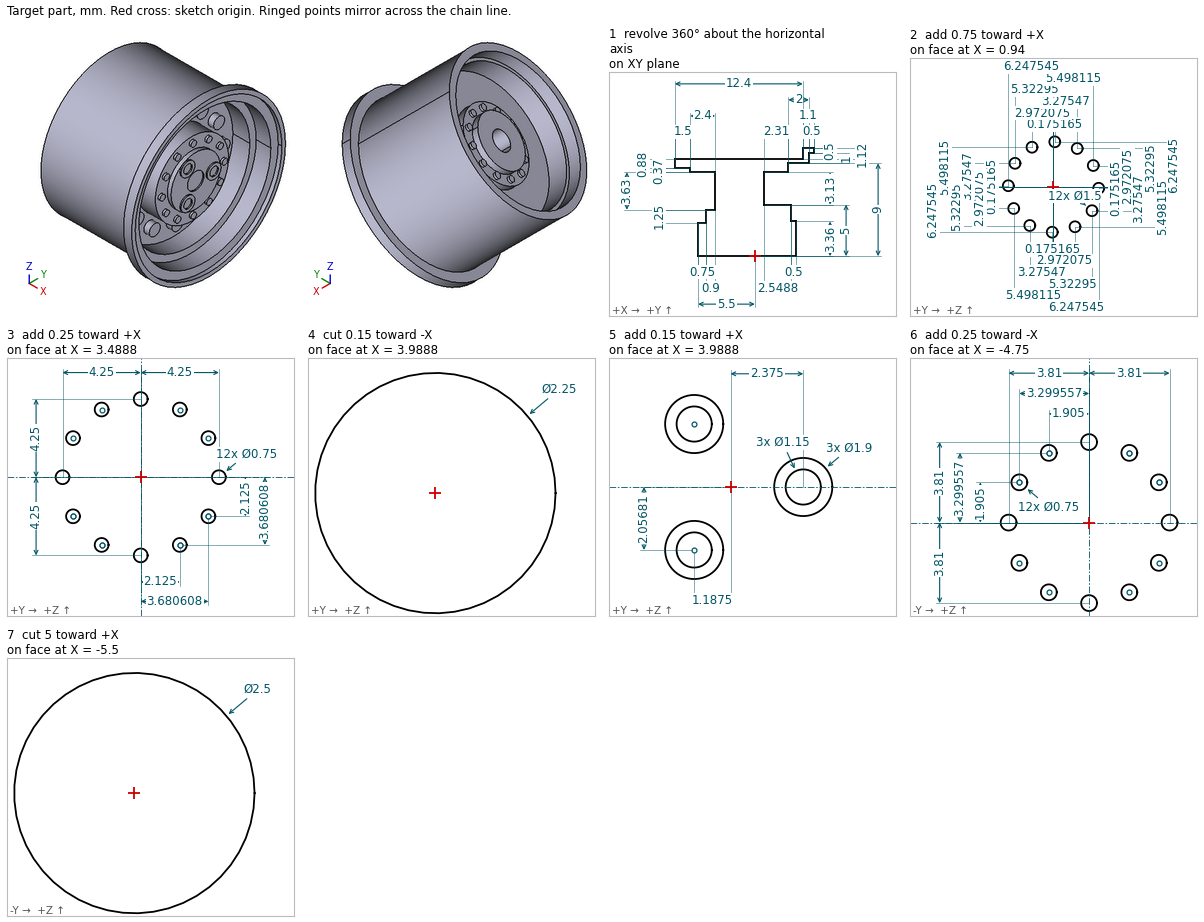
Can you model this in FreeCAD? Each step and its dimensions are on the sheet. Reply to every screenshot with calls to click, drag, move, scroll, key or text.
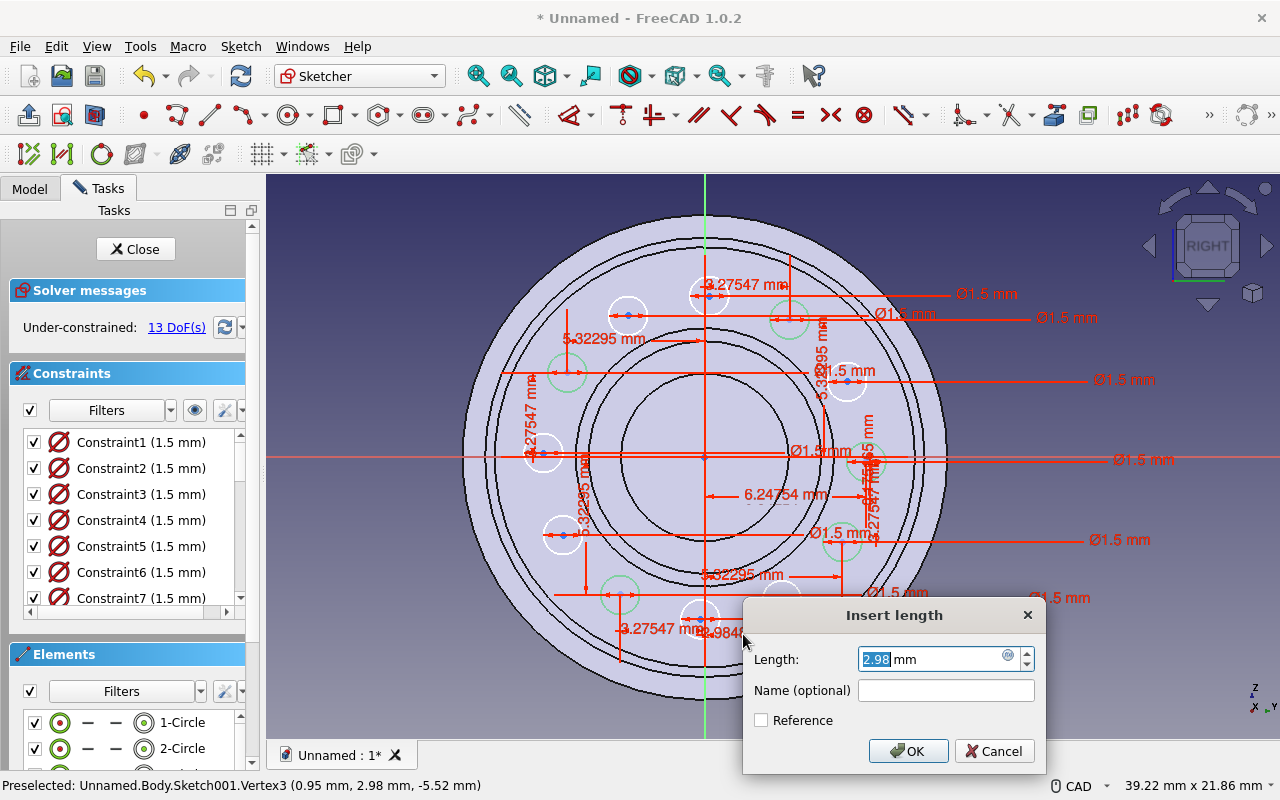
text(2.972075)
key(Return)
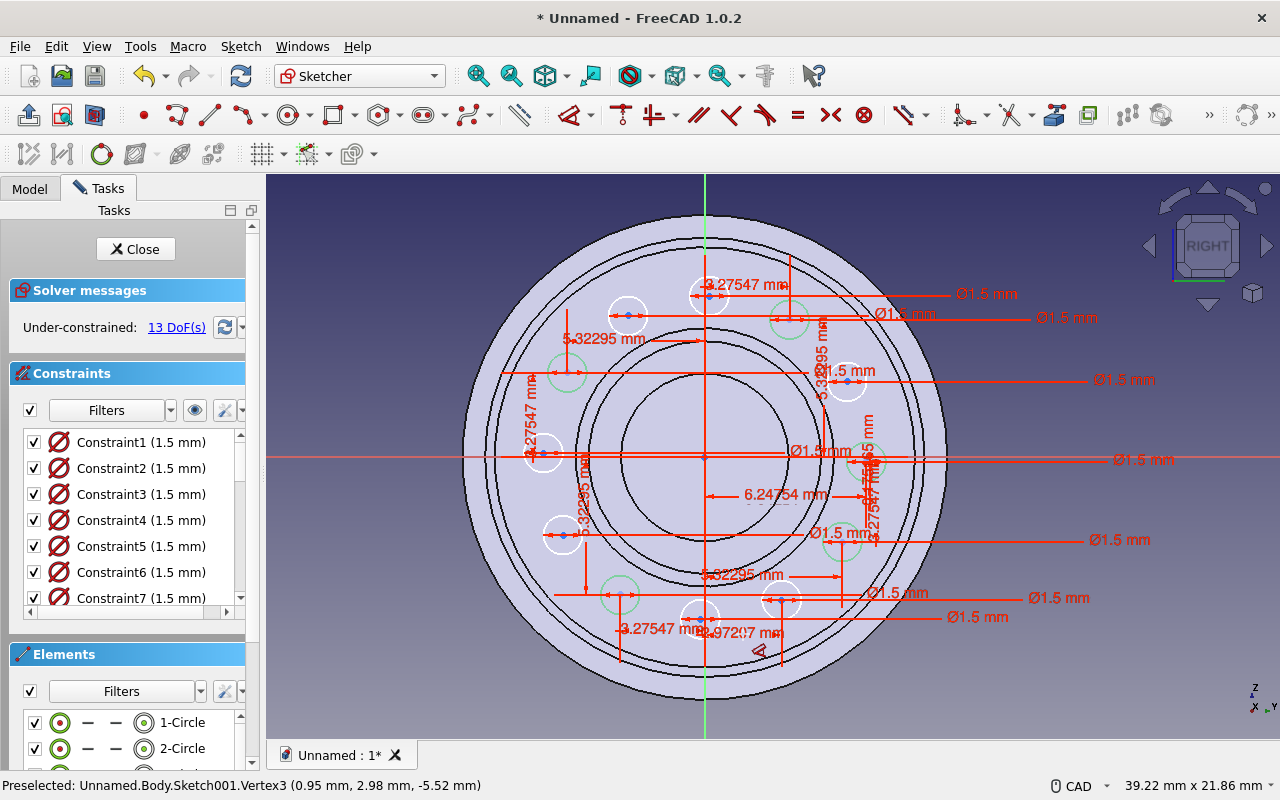
click(782, 600)
click(816, 562)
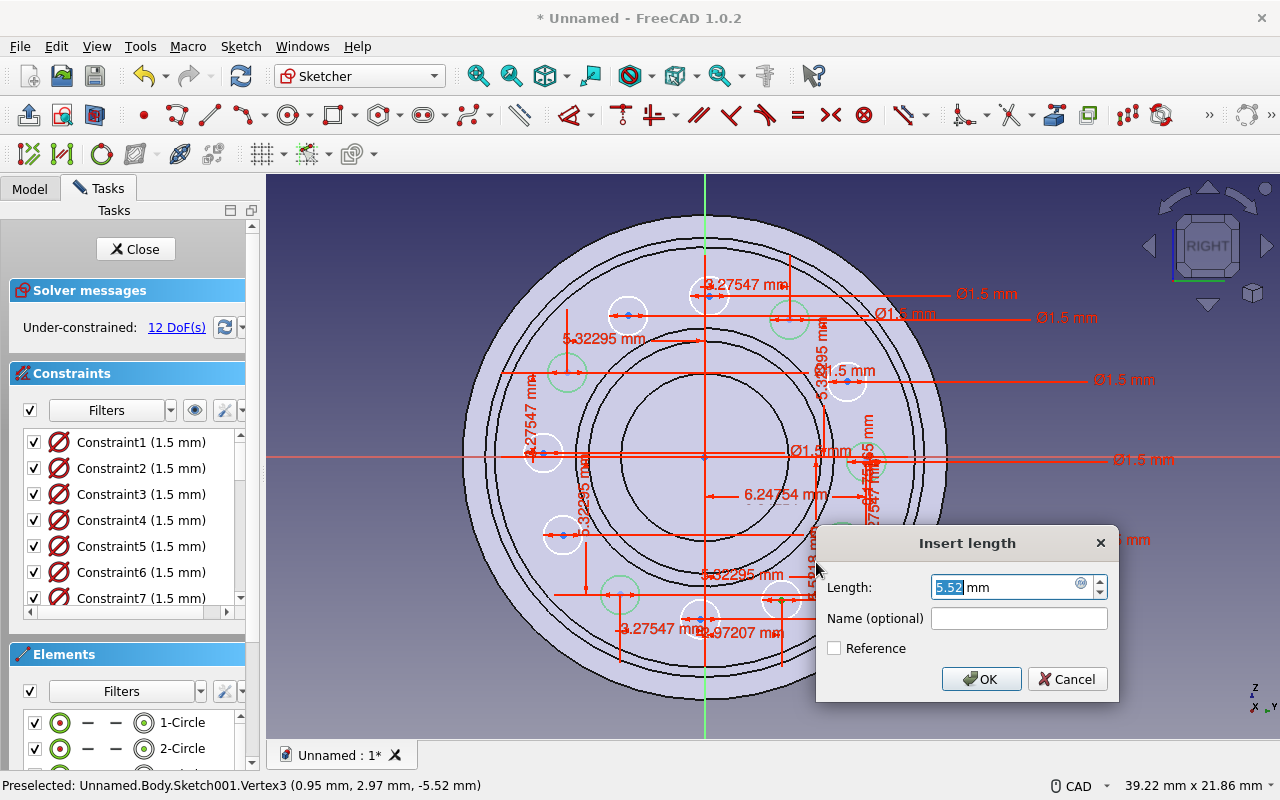
text(5.498115)
key(Return)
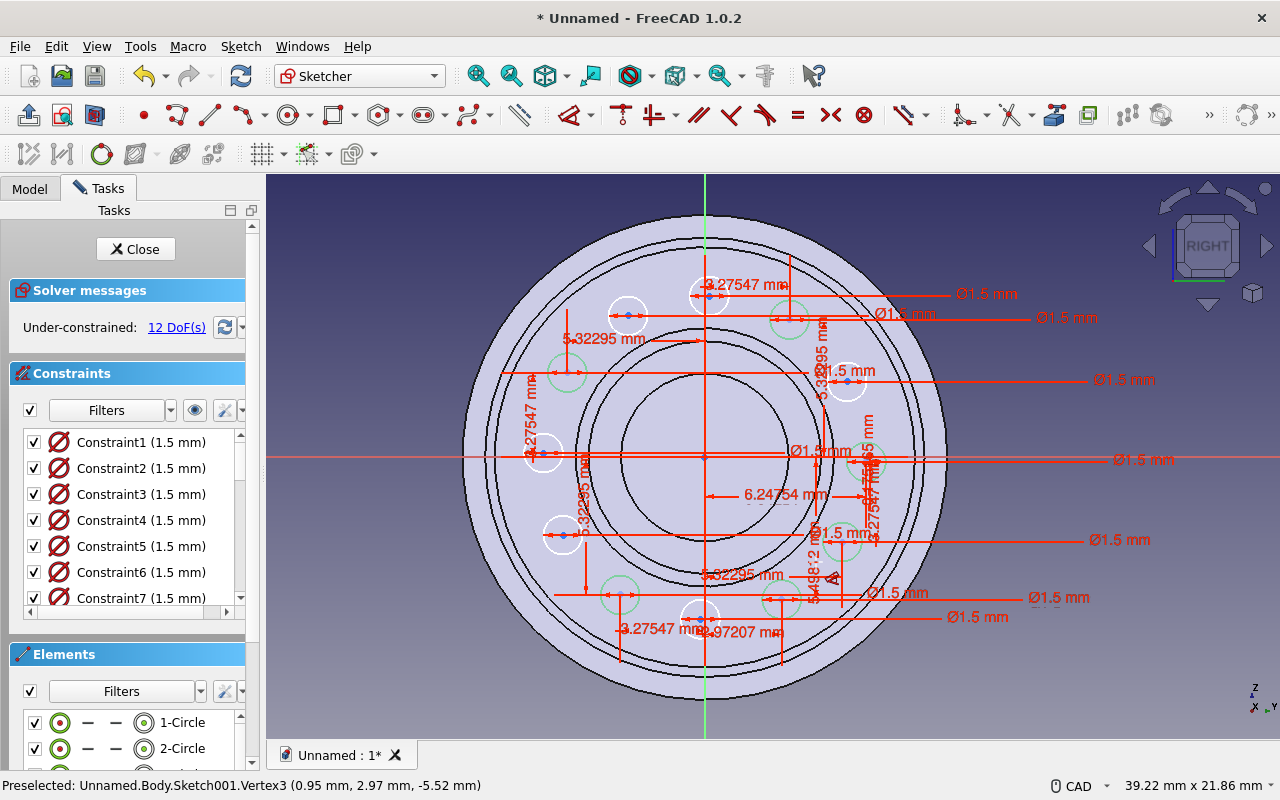
scroll(700, 619, up, 11)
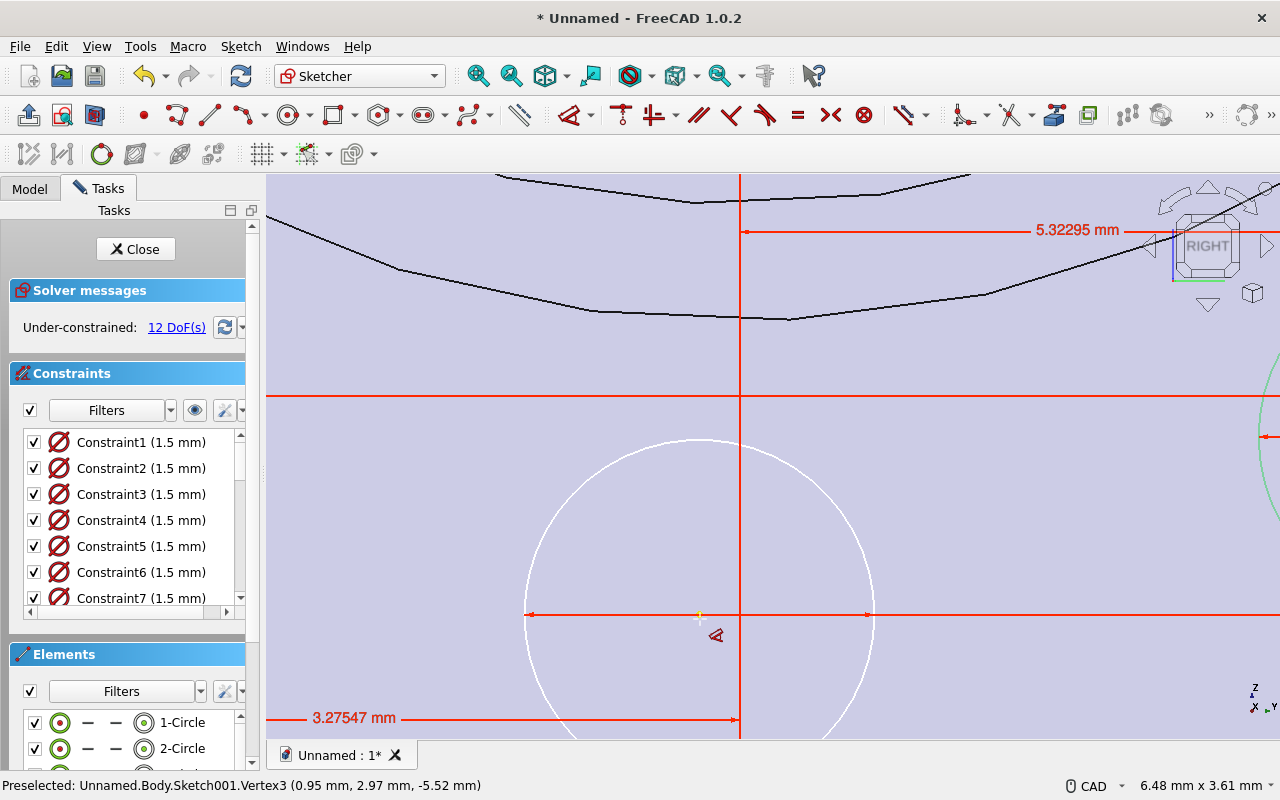
click(699, 615)
click(720, 649)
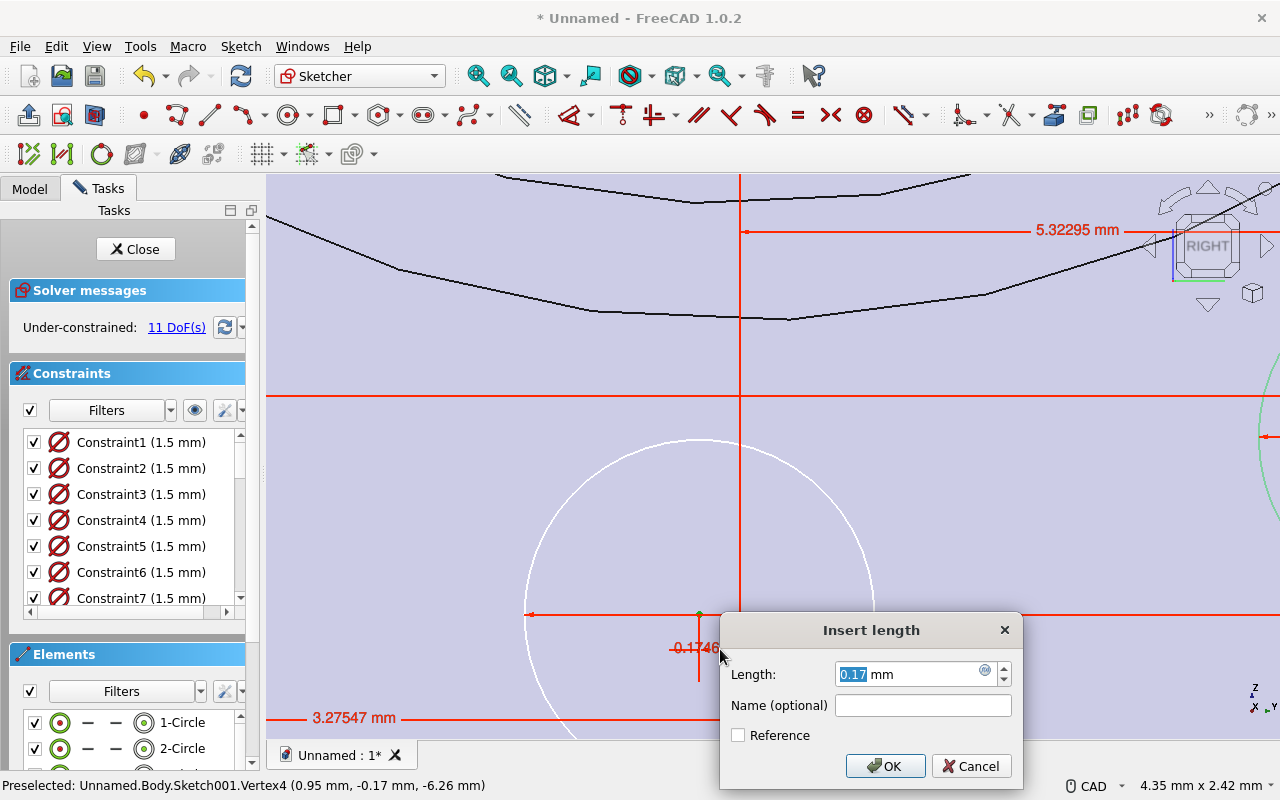
text(0.175165)
key(Return)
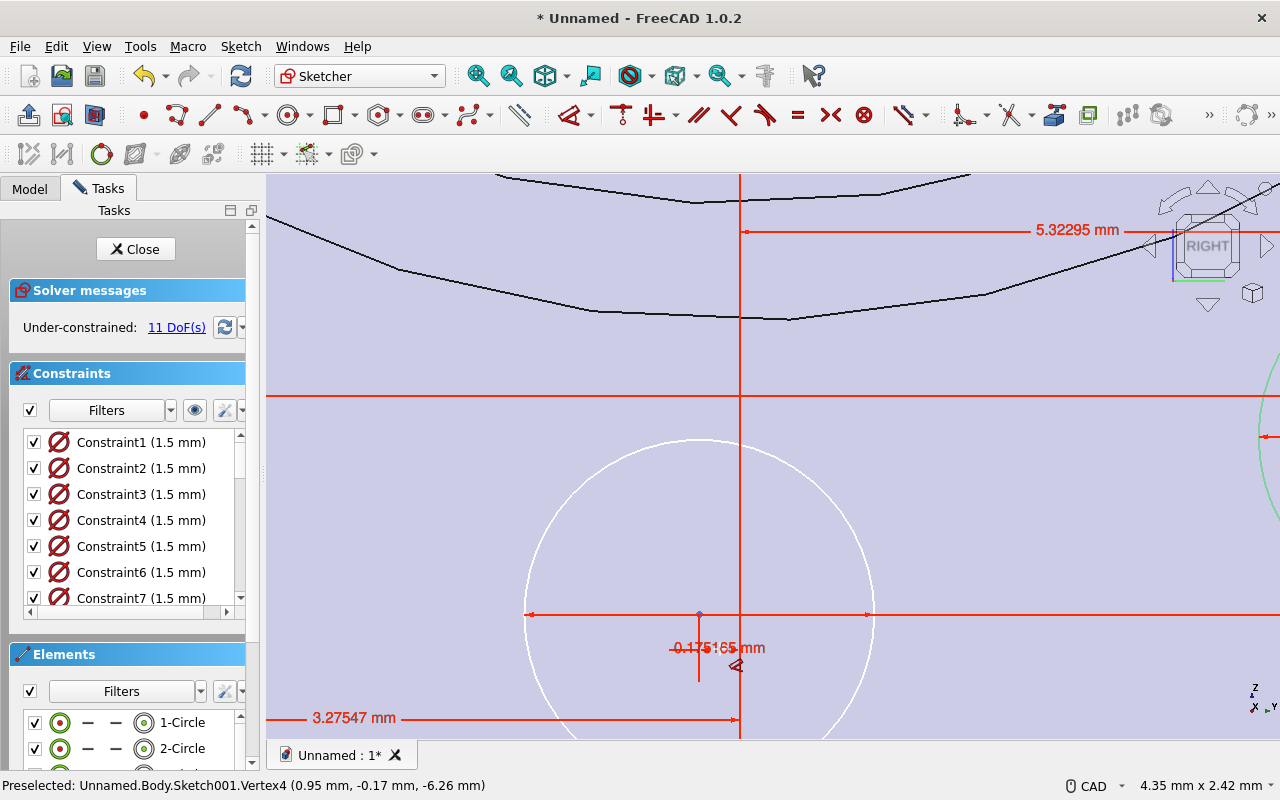
scroll(700, 619, down, 11)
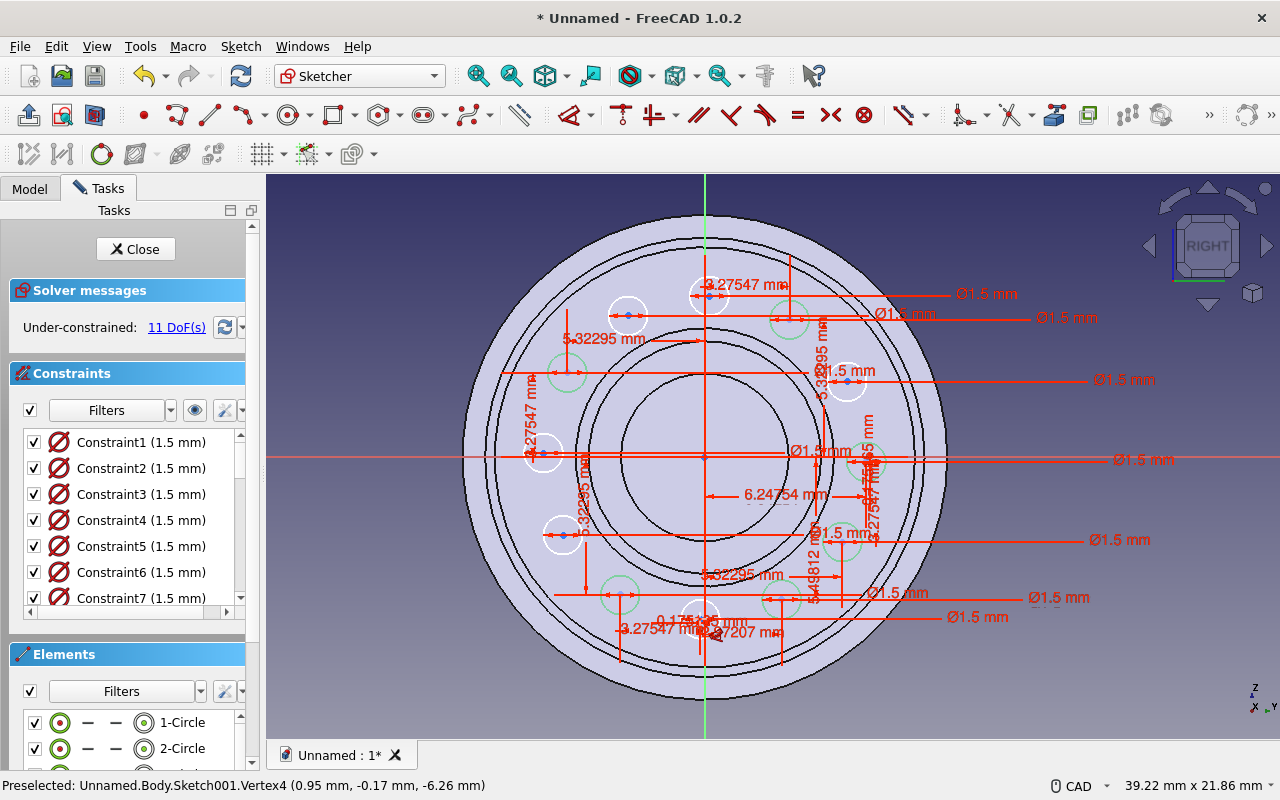
click(700, 619)
click(666, 538)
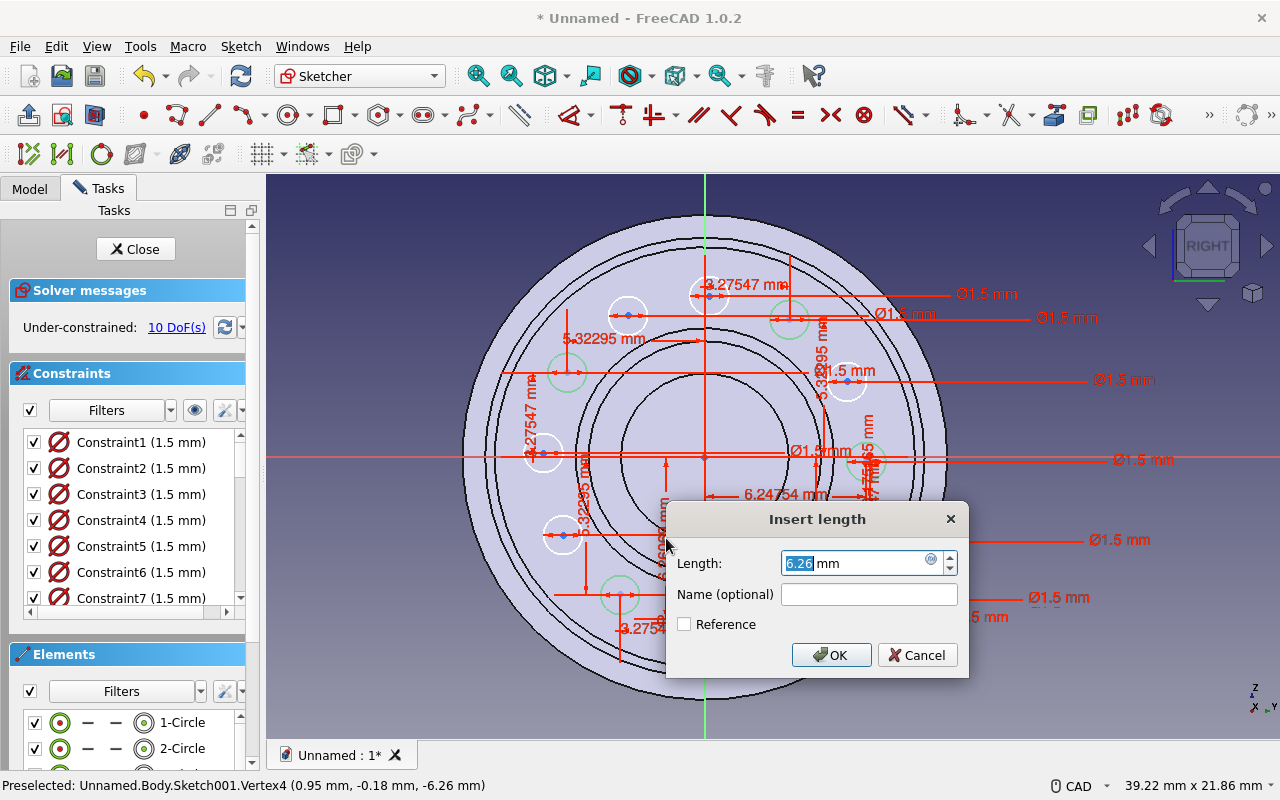
text(6.247545)
key(Return)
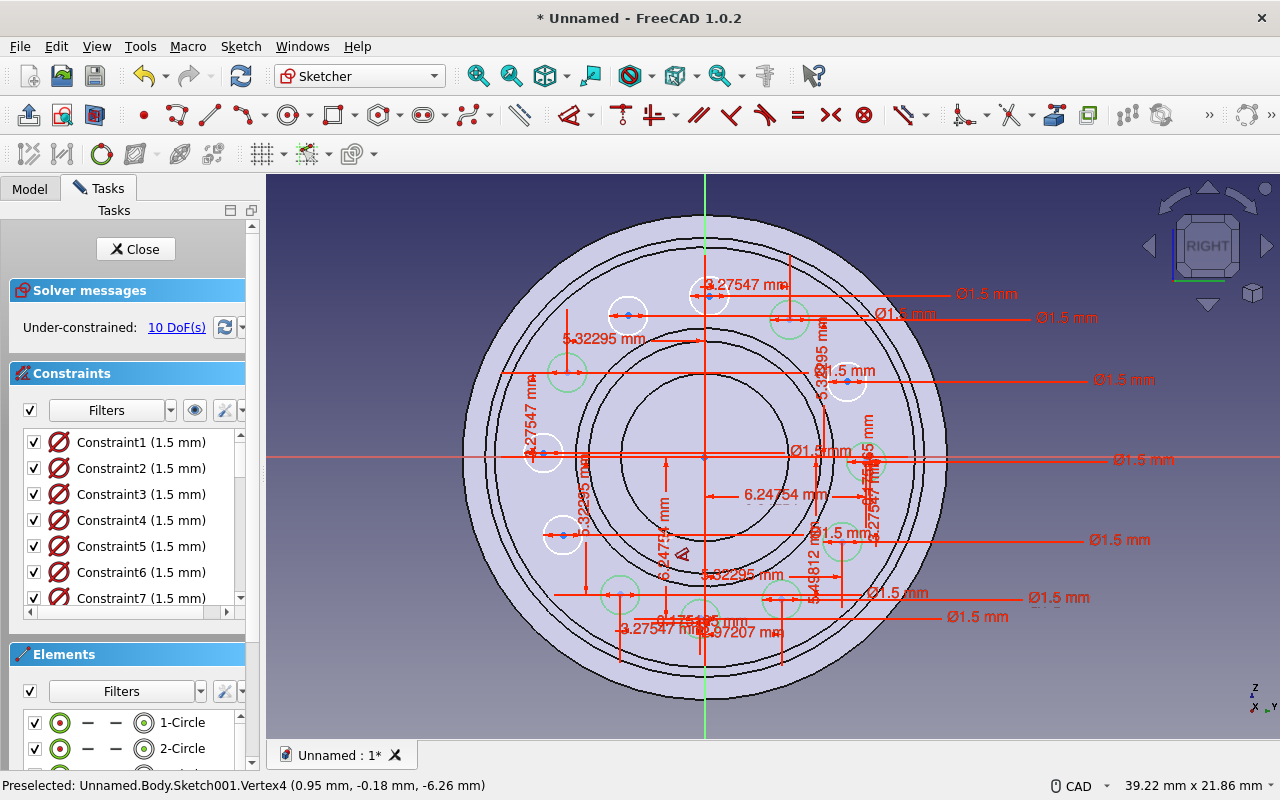
click(563, 535)
click(667, 569)